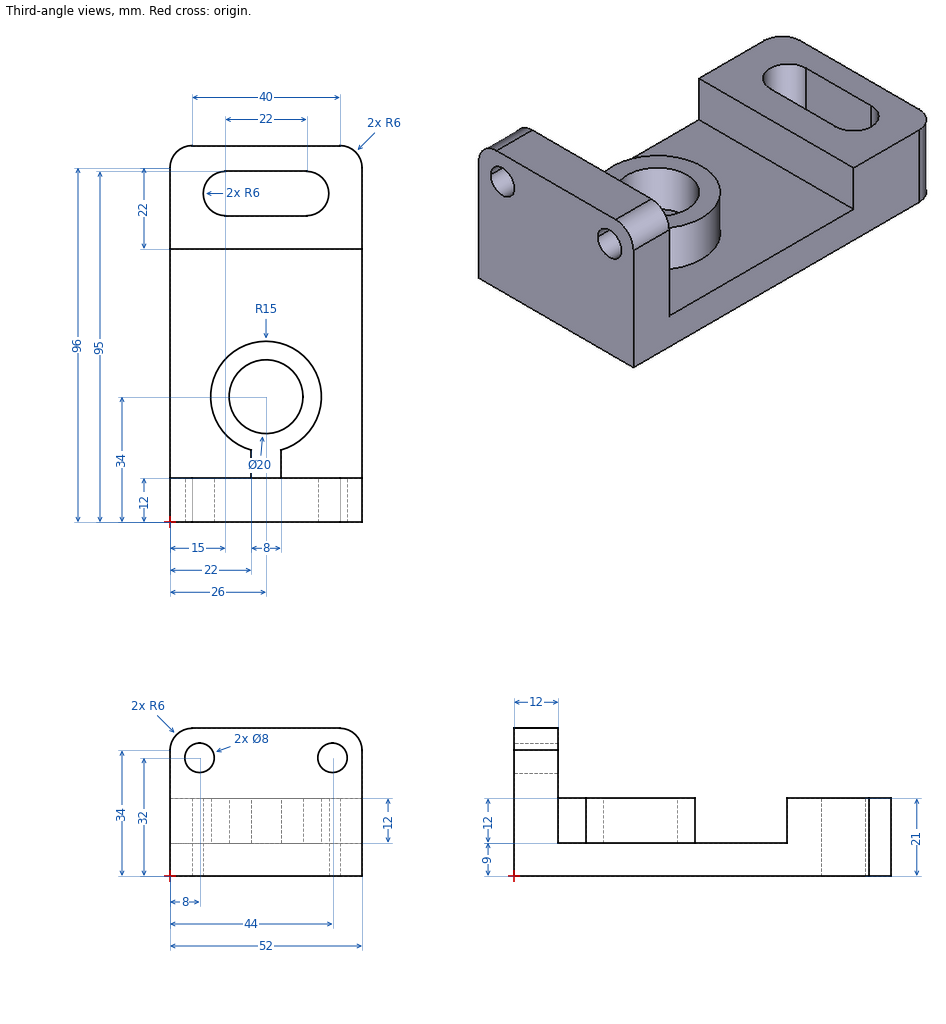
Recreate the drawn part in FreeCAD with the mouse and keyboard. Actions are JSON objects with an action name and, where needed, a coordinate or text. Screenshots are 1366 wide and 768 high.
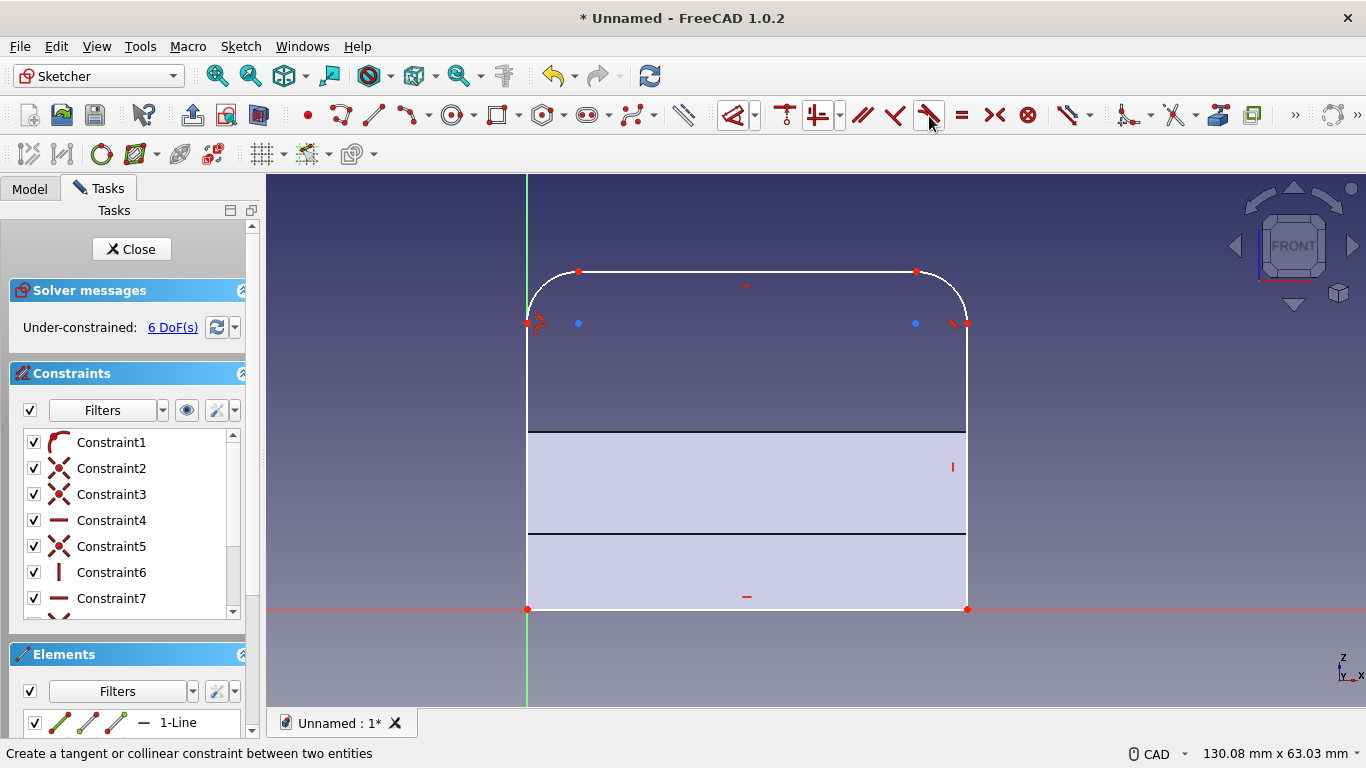
{"action": "left_click", "coordinate": [815, 272]}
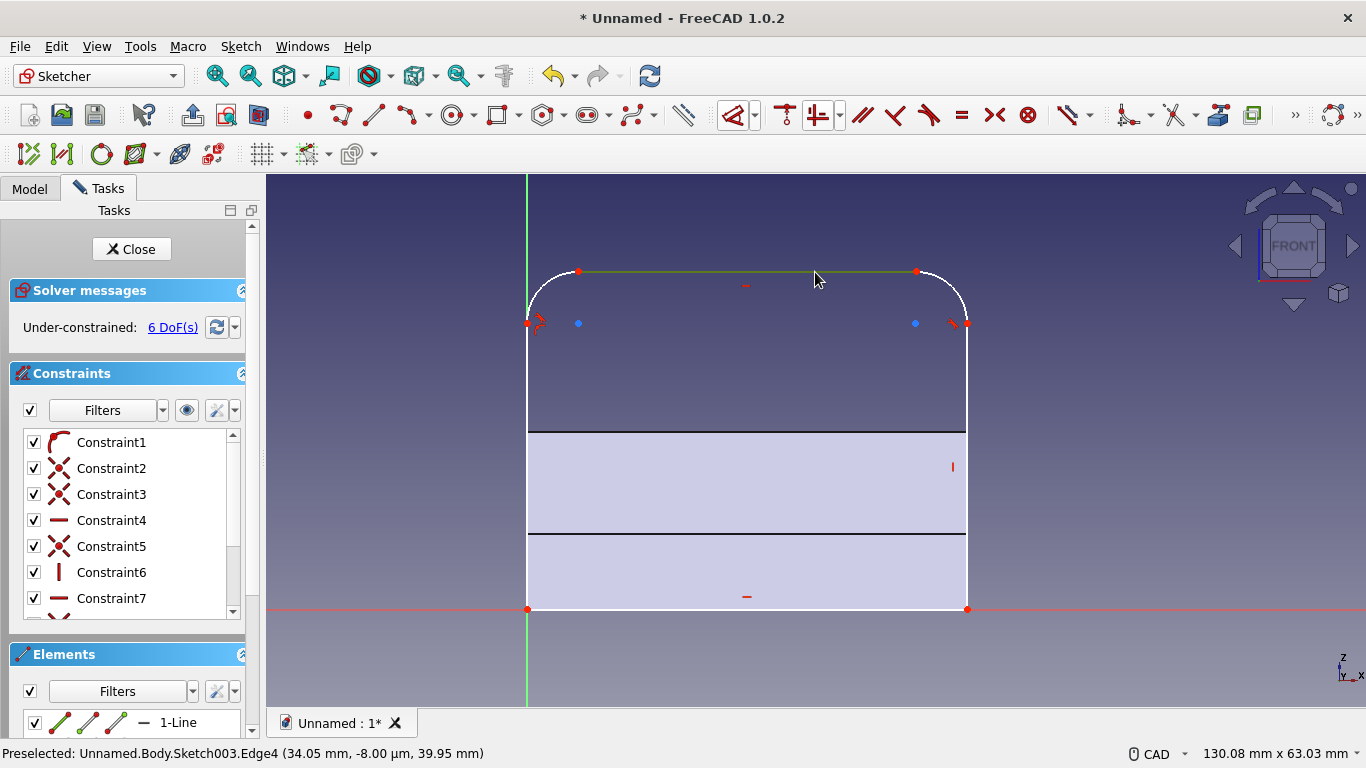
{"action": "left_click", "coordinate": [962, 300]}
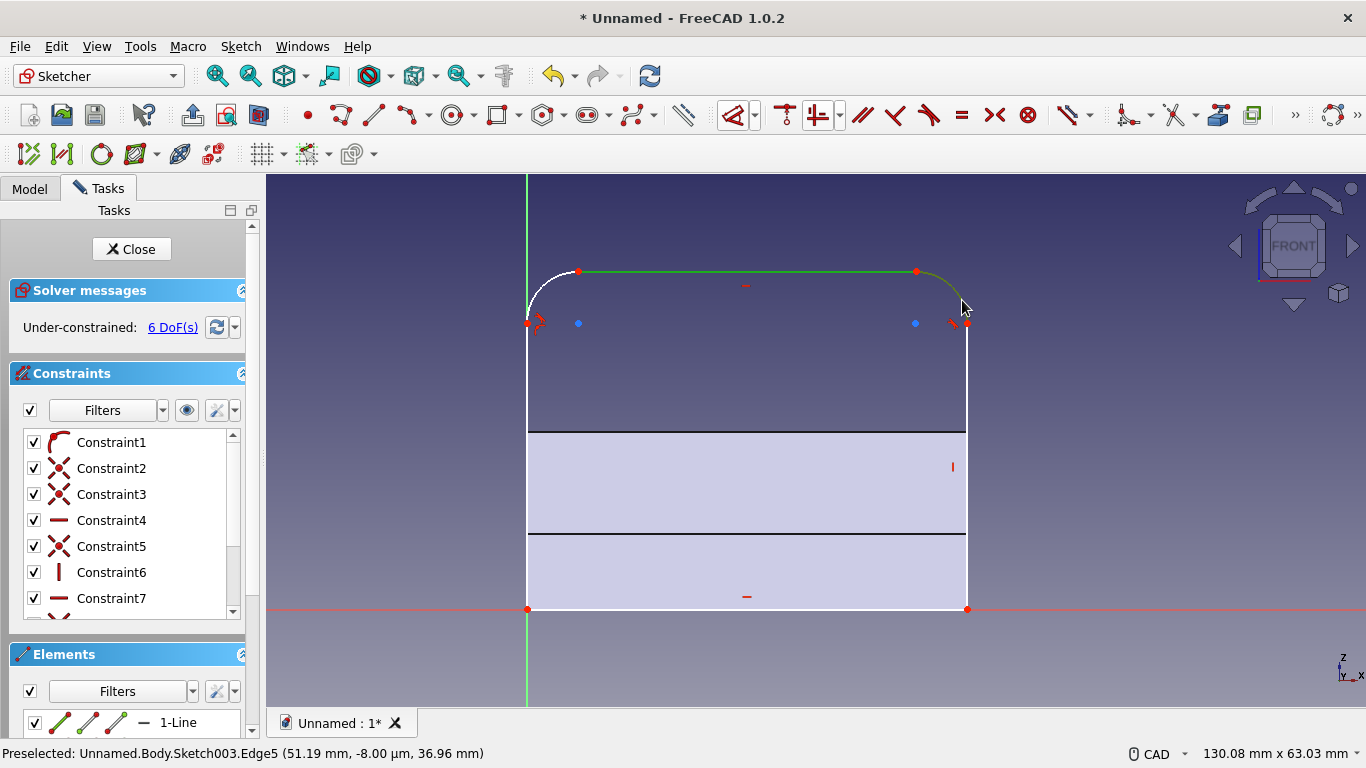
{"action": "left_click", "coordinate": [929, 116]}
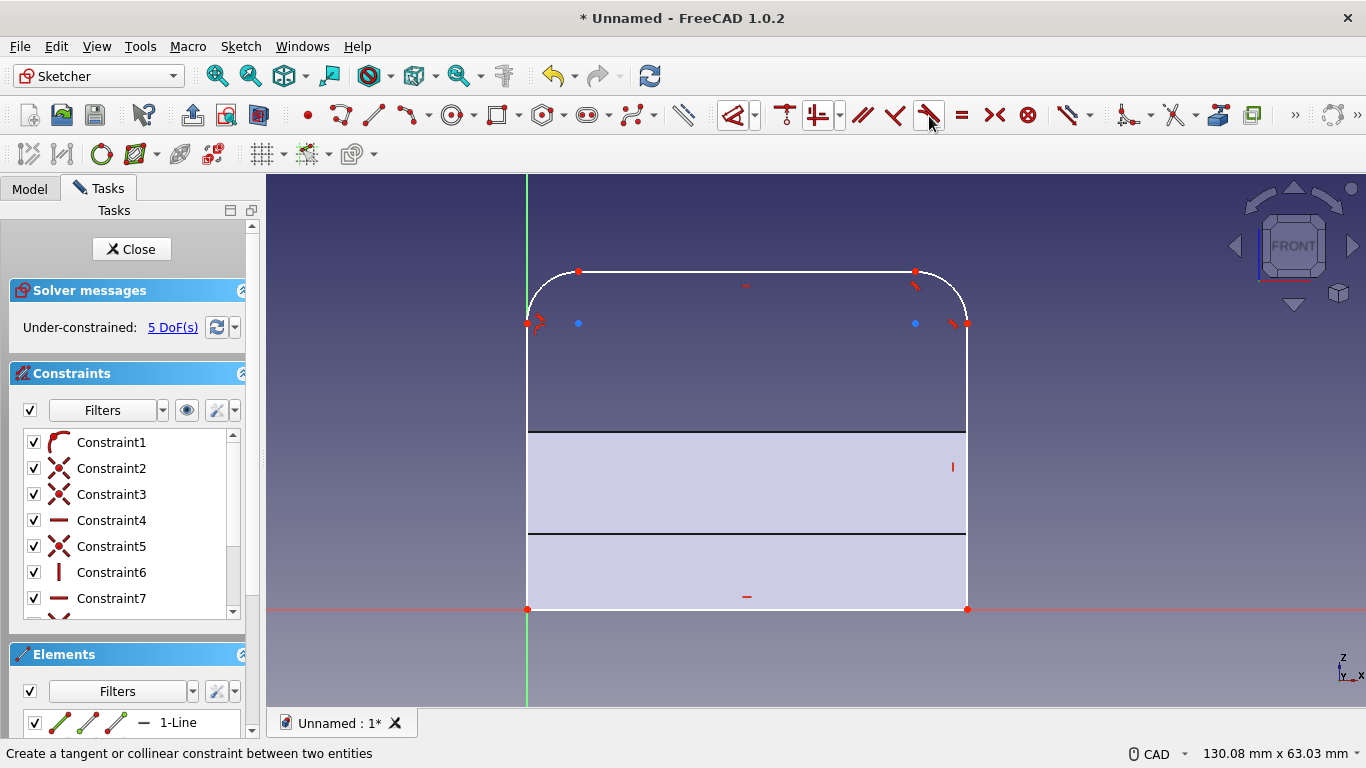
{"action": "left_click", "coordinate": [814, 272]}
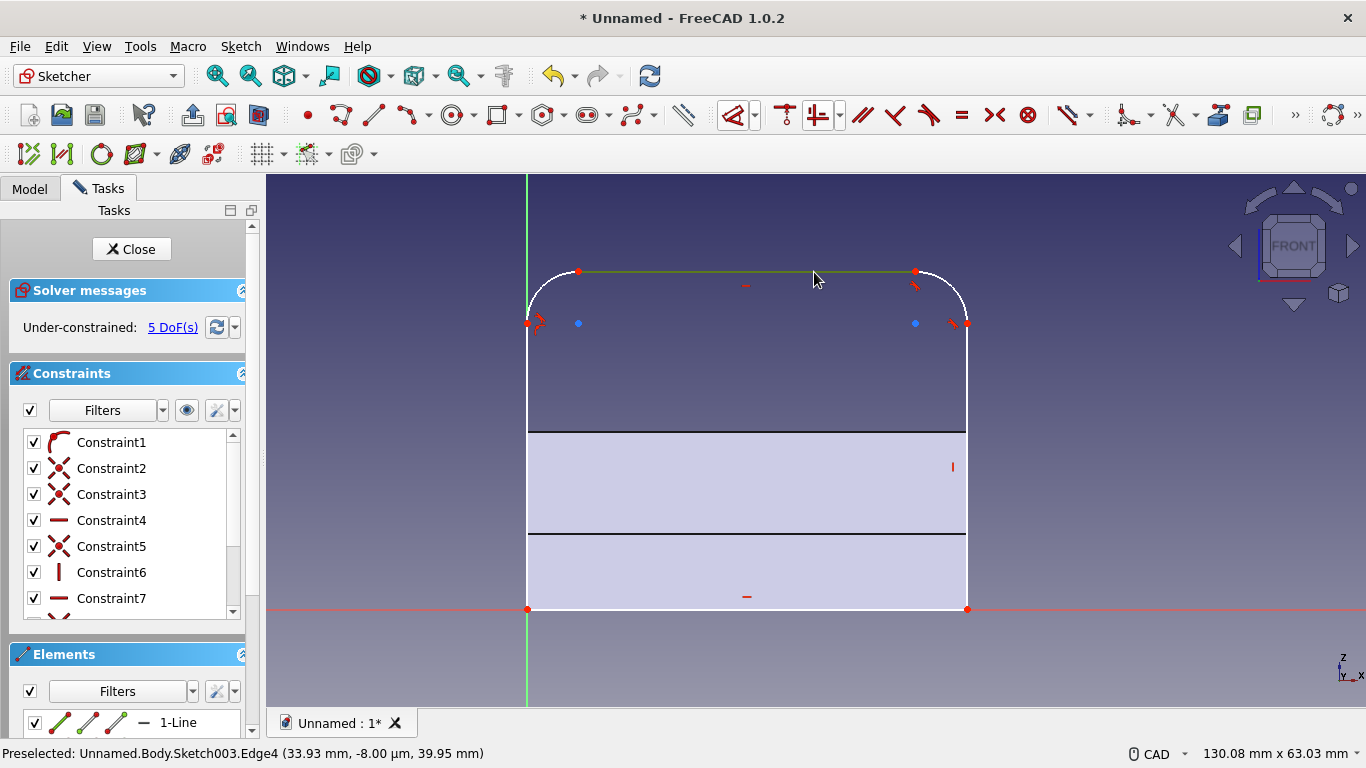
{"action": "left_click", "coordinate": [555, 278]}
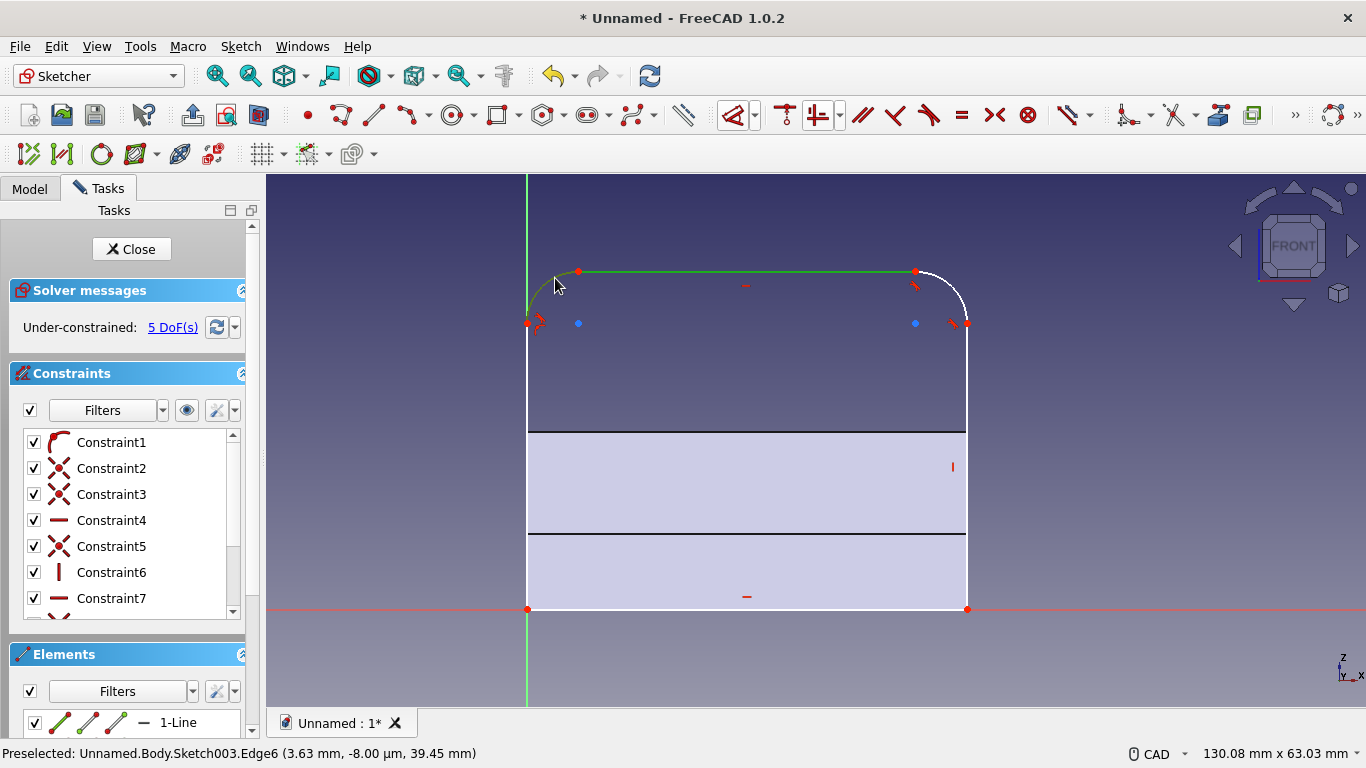
{"action": "key", "text": "t"}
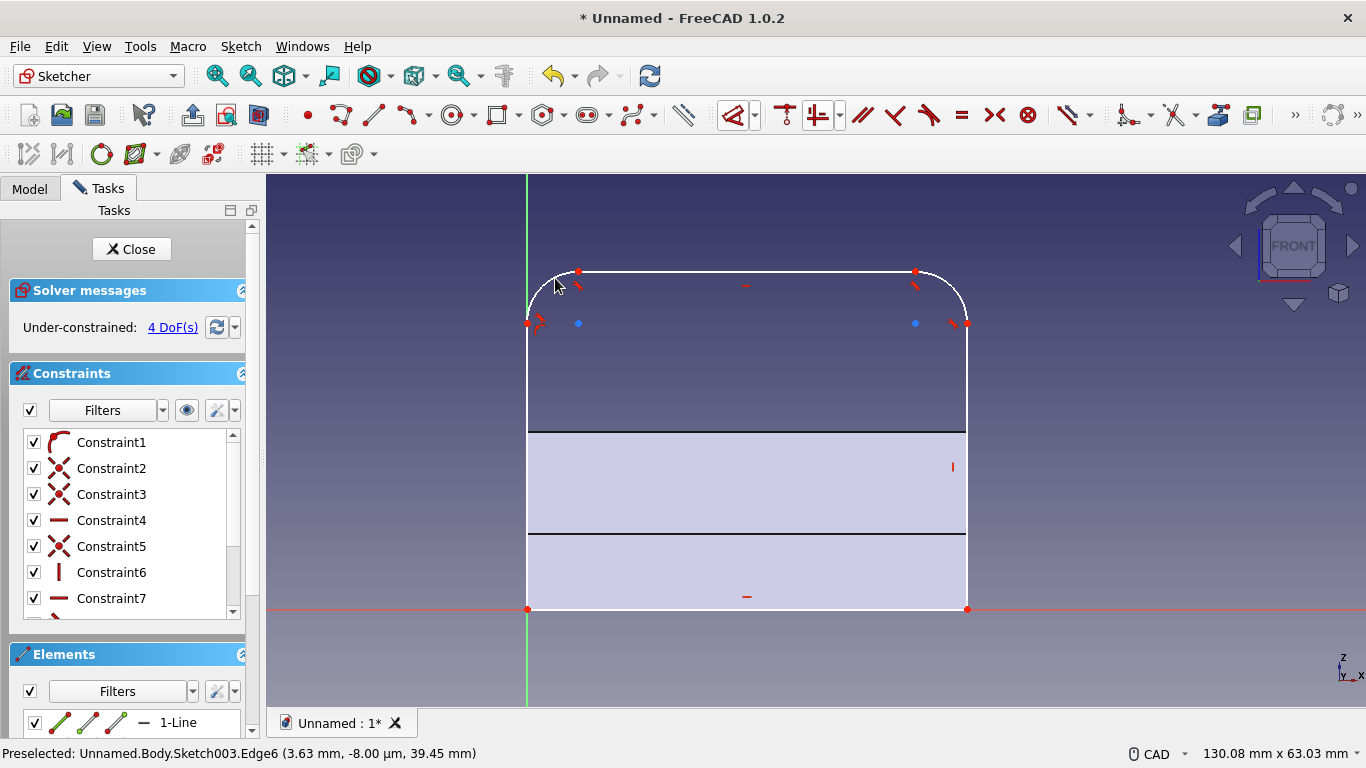
{"action": "left_click", "coordinate": [961, 300]}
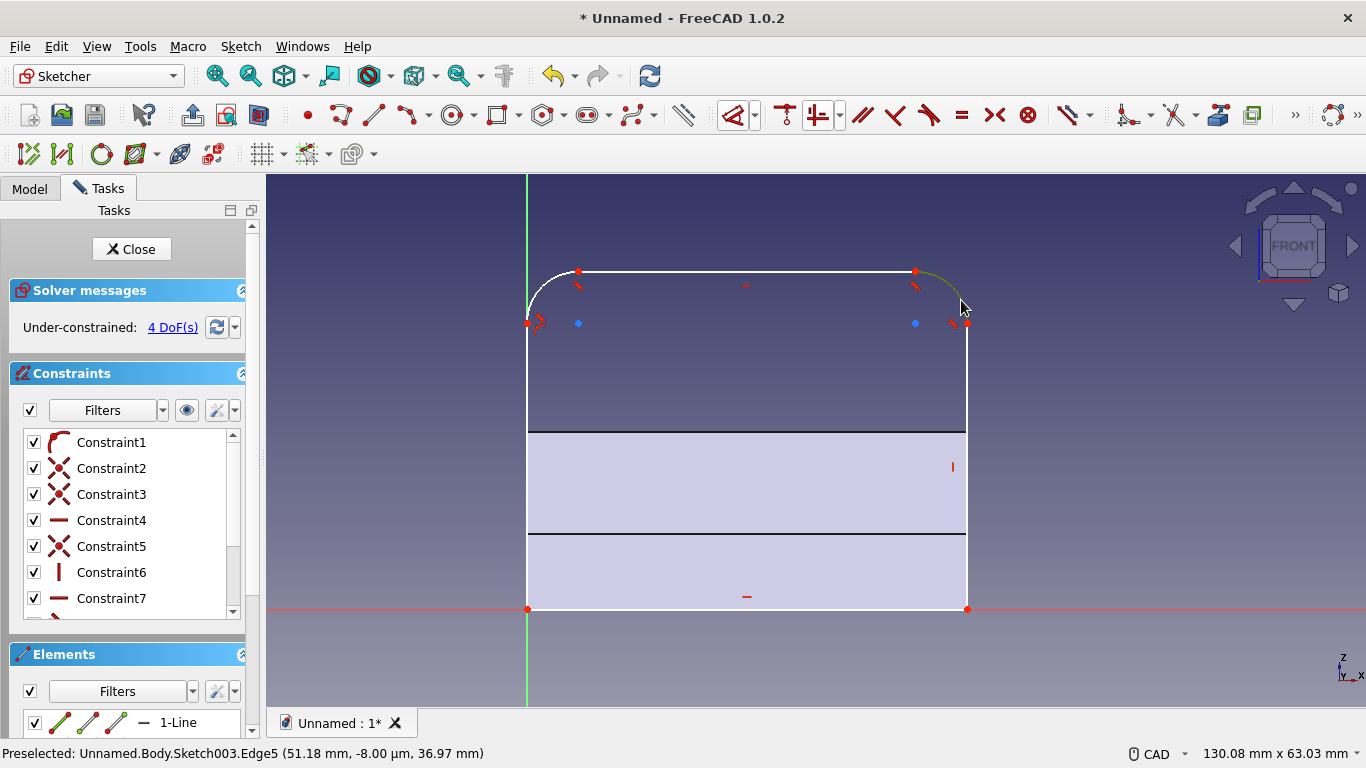
{"action": "left_click", "coordinate": [555, 277]}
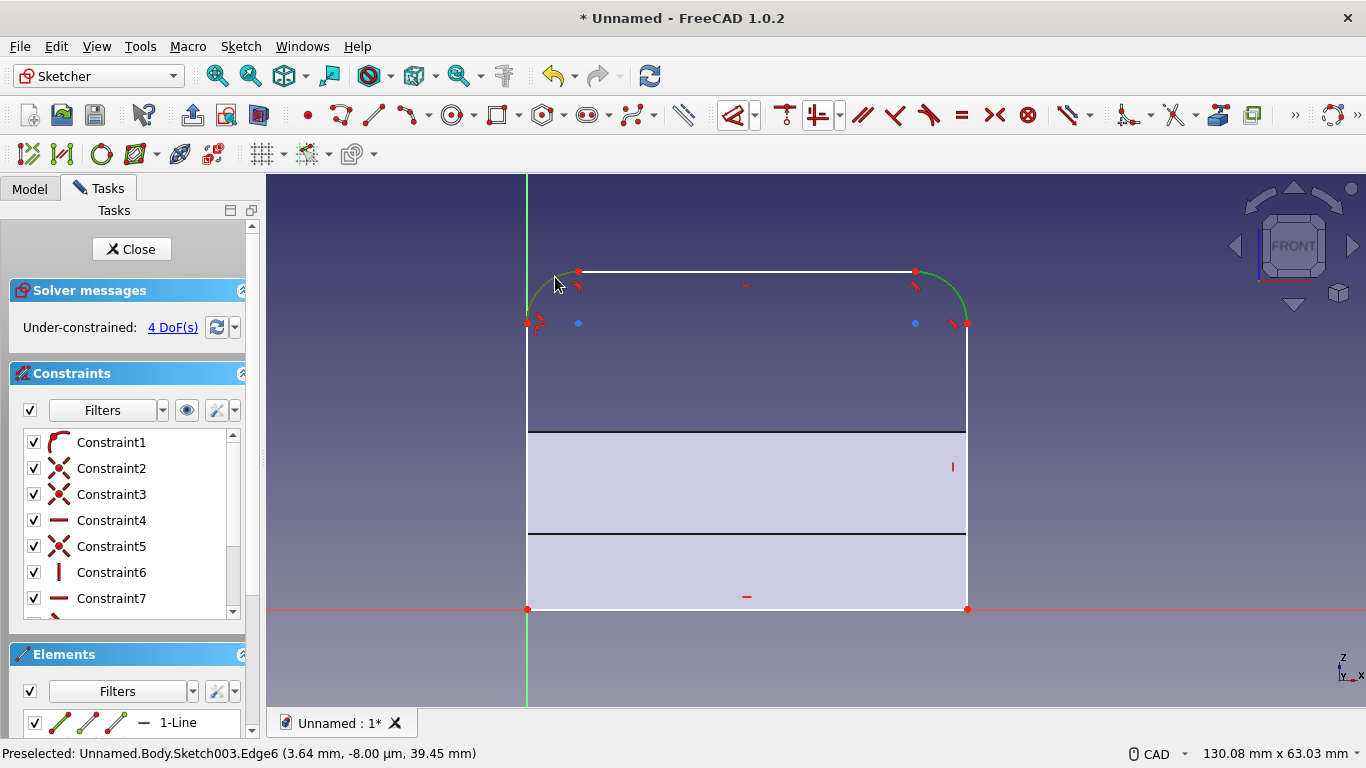
{"action": "left_click", "coordinate": [962, 116]}